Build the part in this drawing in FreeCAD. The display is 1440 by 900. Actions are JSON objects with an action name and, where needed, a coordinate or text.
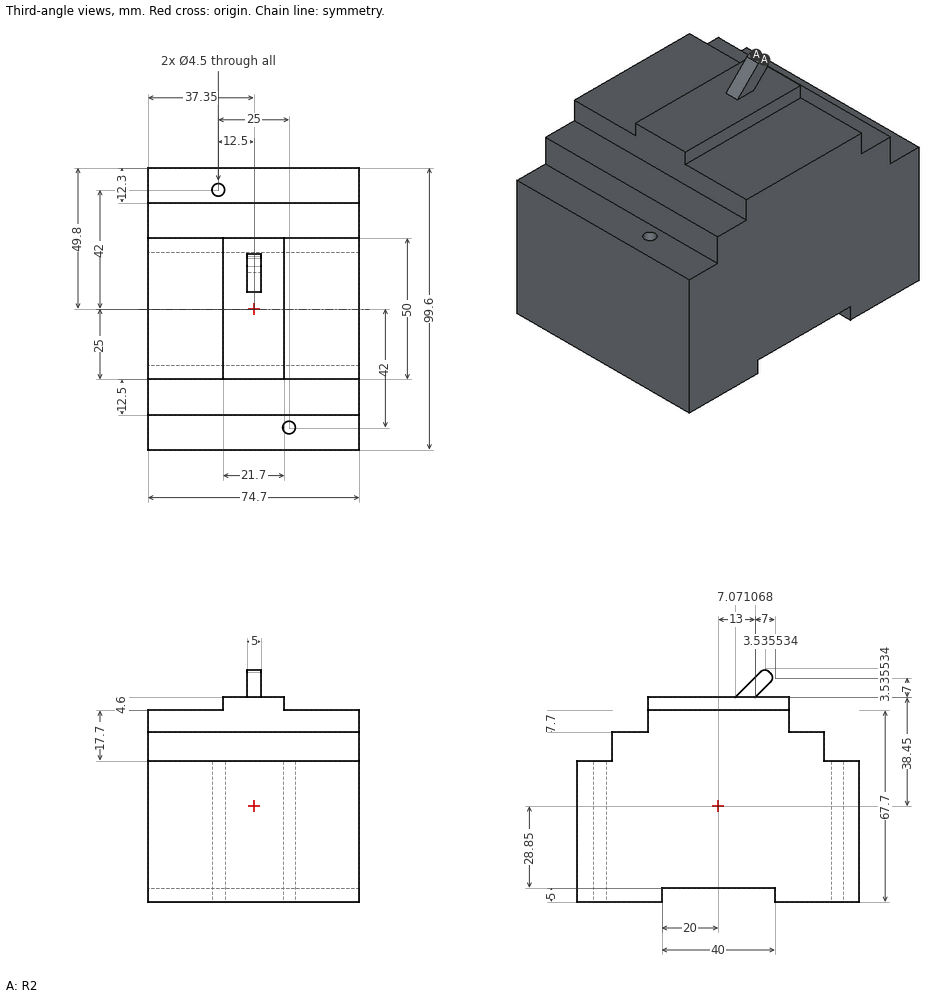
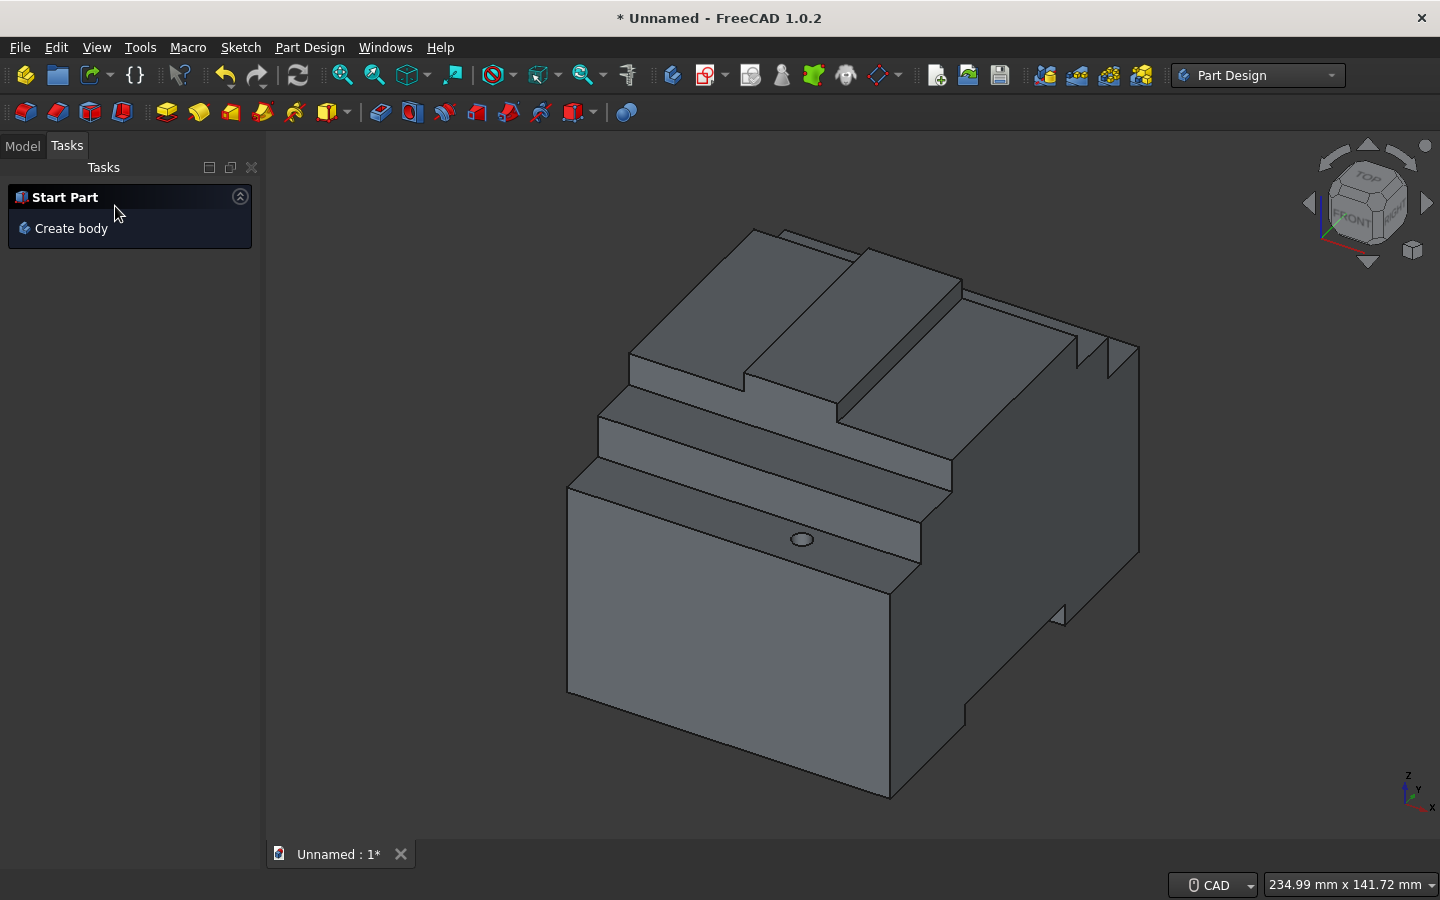
{"action": "left_click", "coordinate": [706, 76]}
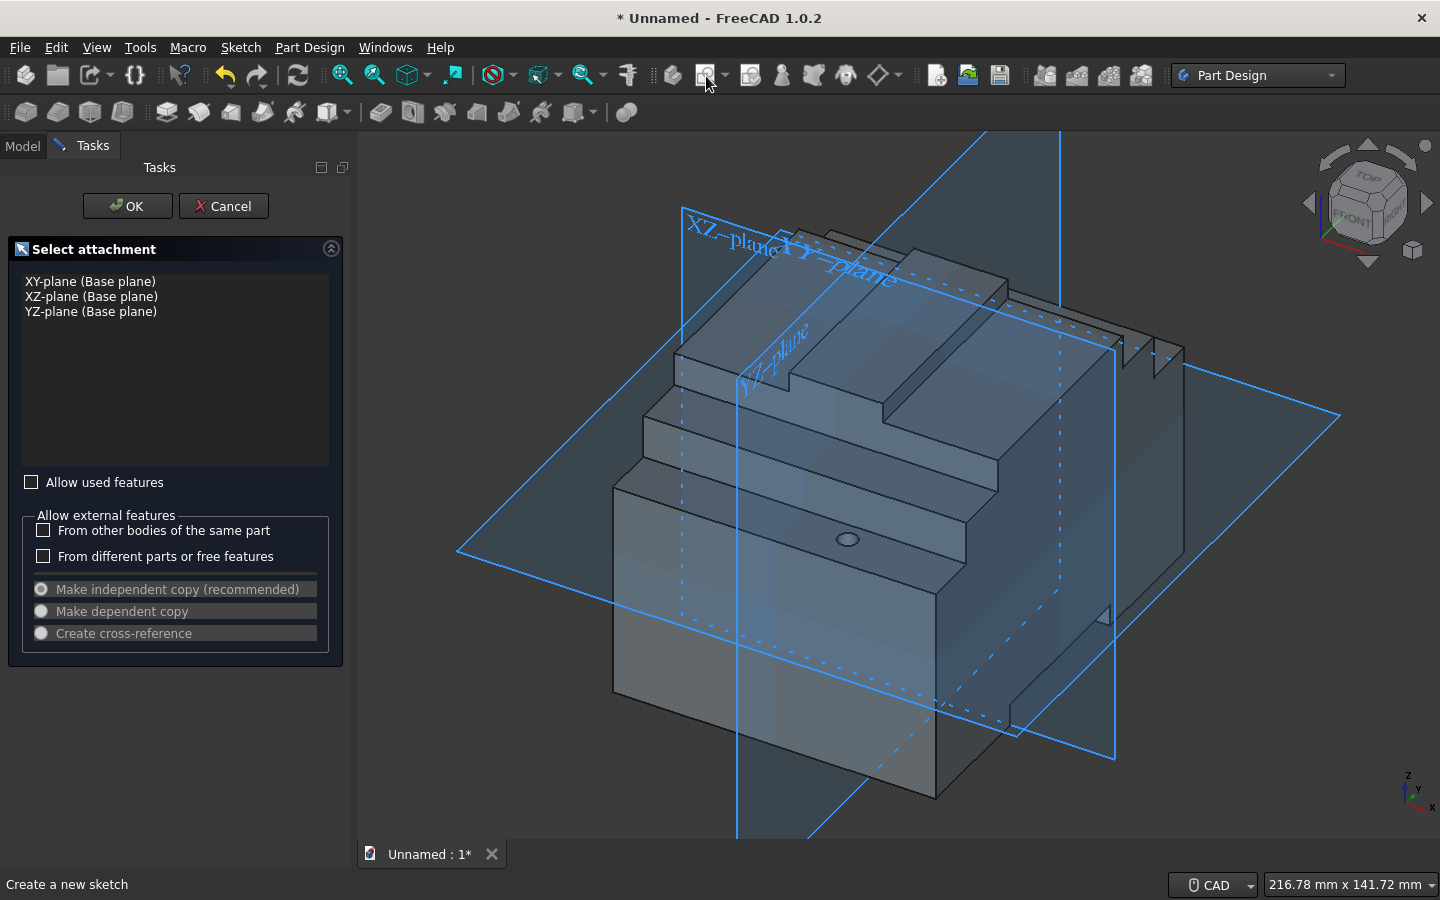
{"action": "left_click", "coordinate": [82, 312]}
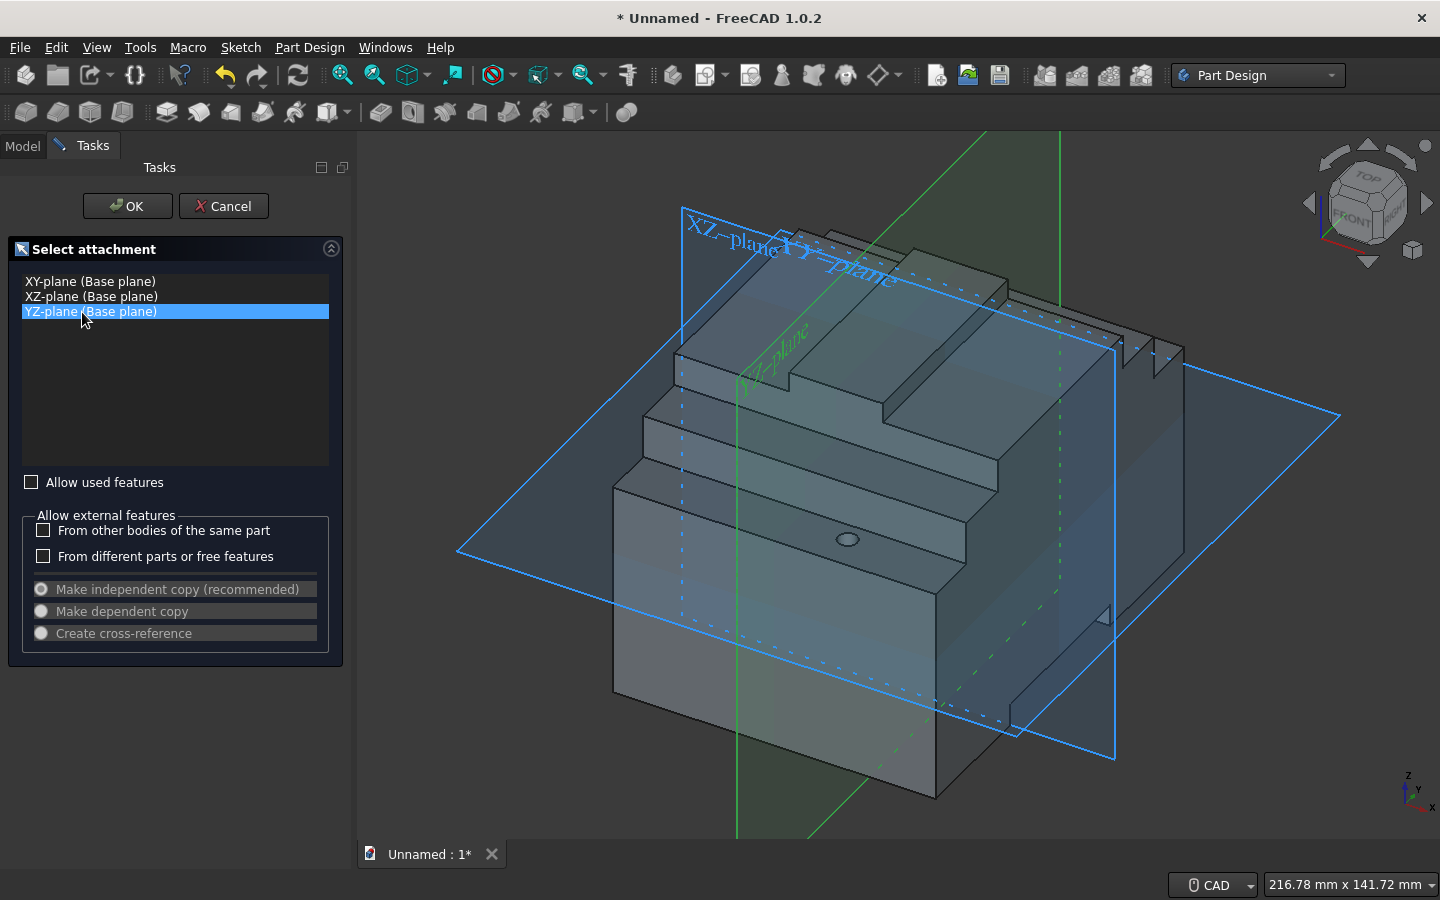
{"action": "left_click", "coordinate": [128, 206]}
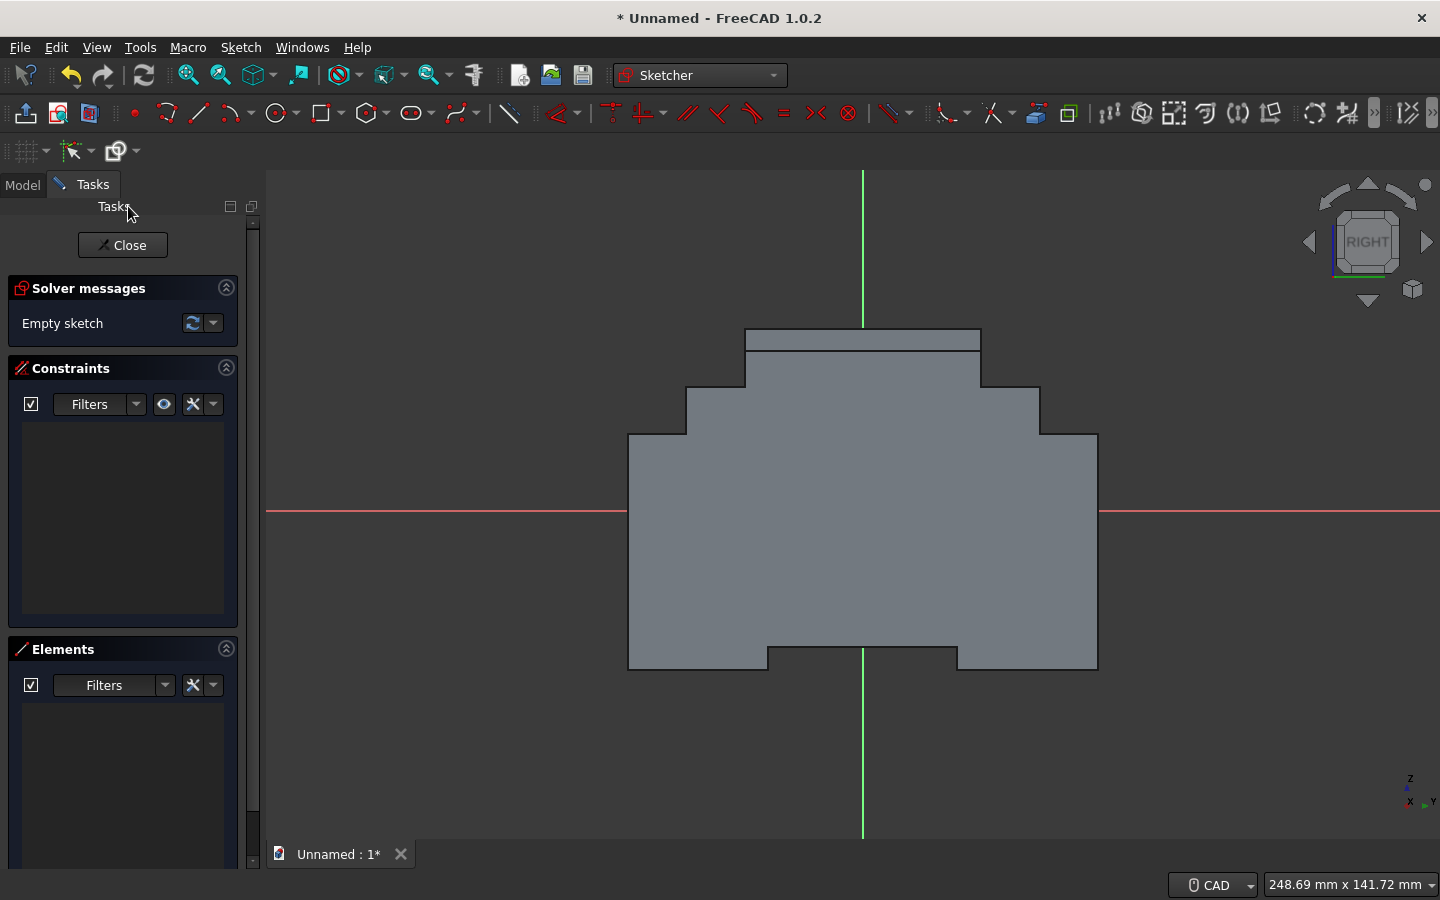
{"action": "left_click", "coordinate": [90, 114]}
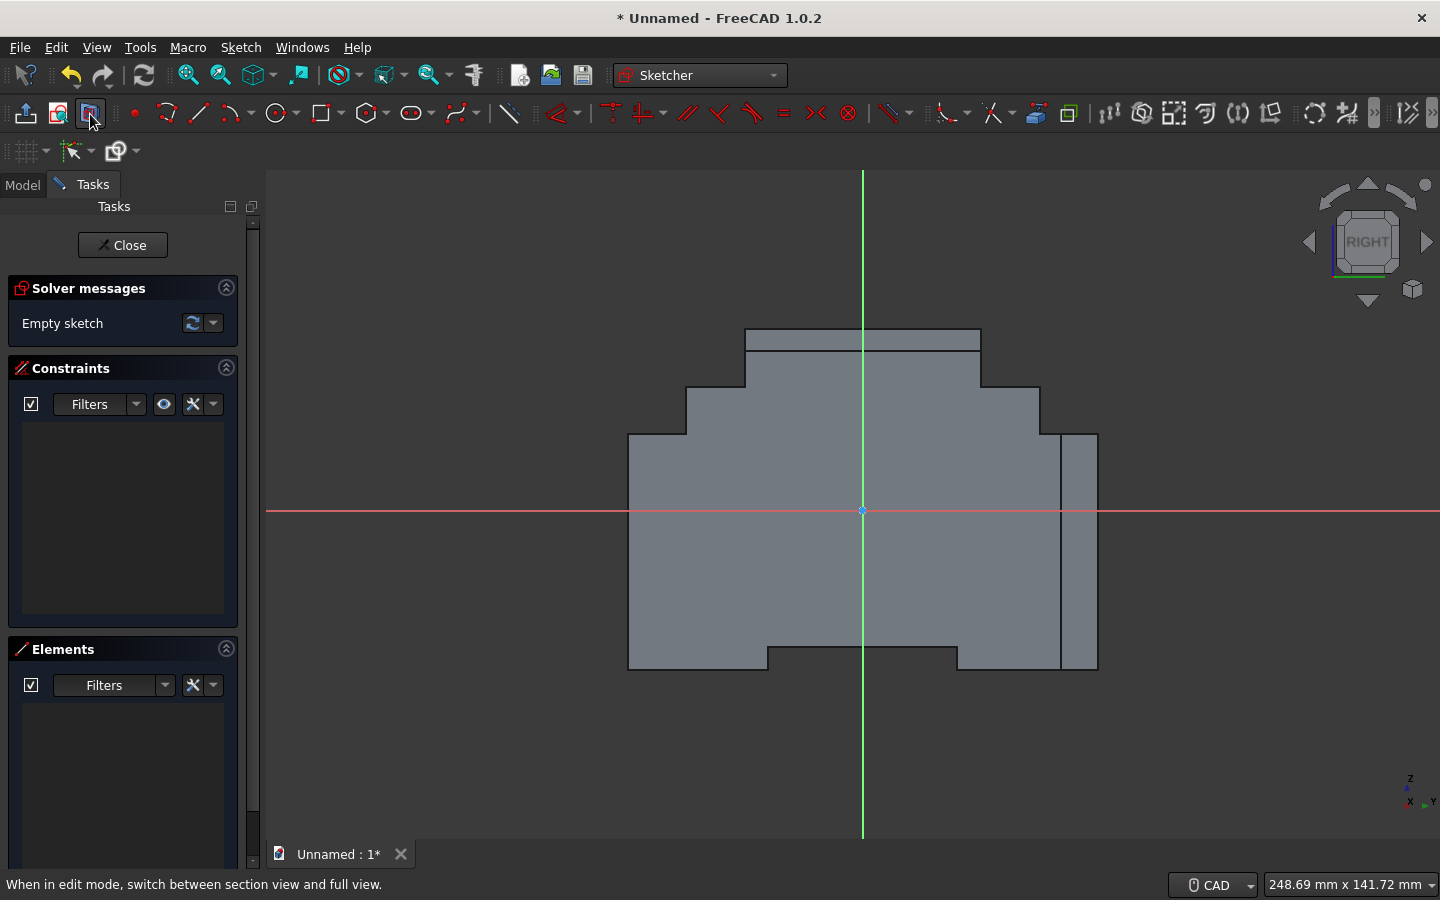
{"action": "scroll", "coordinate": [941, 279], "scroll_direction": "up", "scroll_amount": 11}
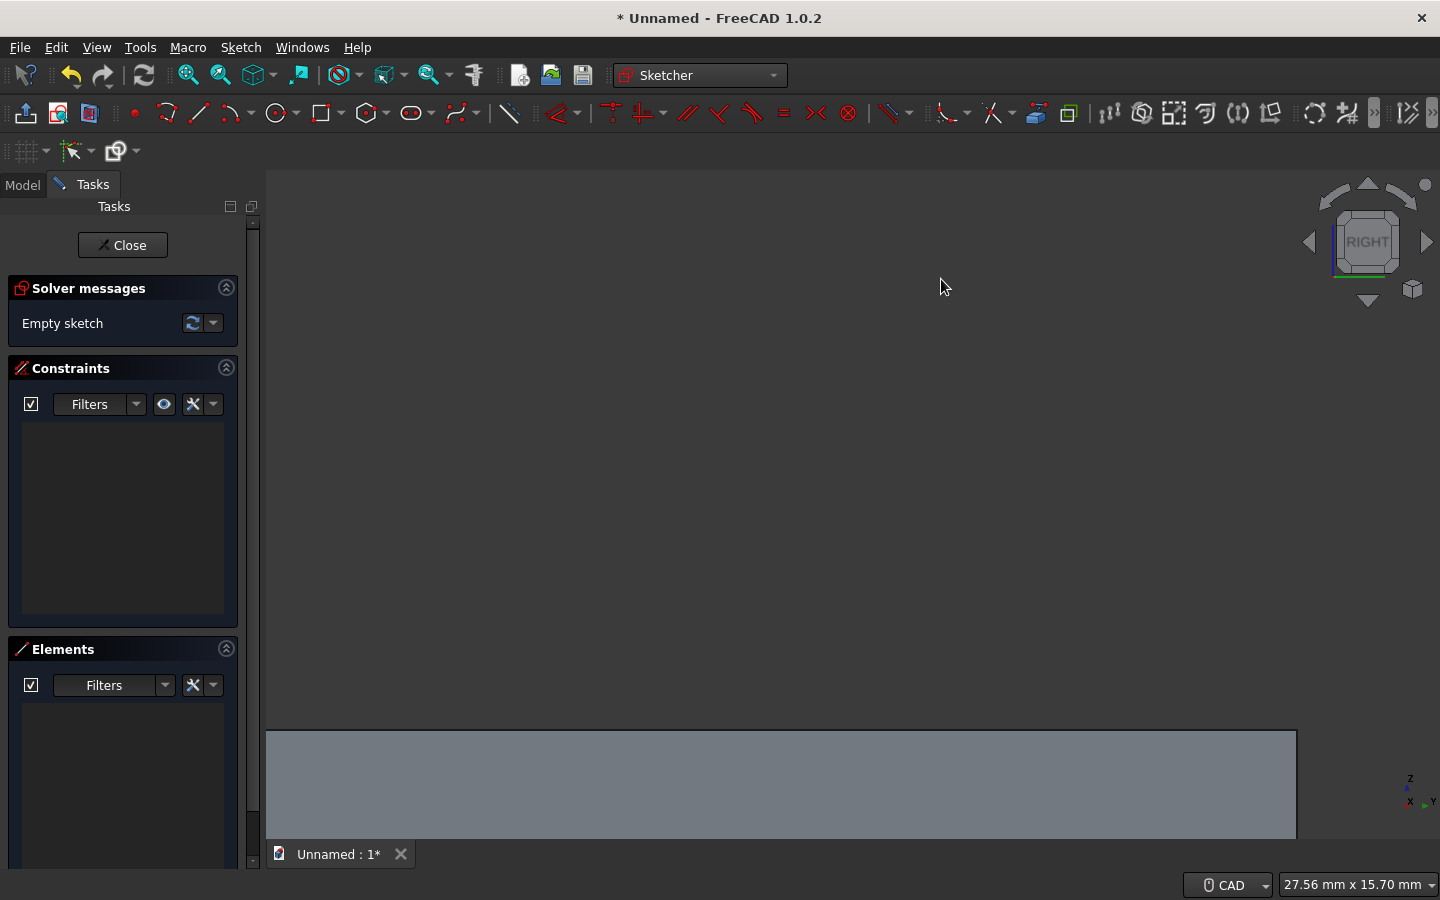
{"action": "left_click", "coordinate": [168, 114]}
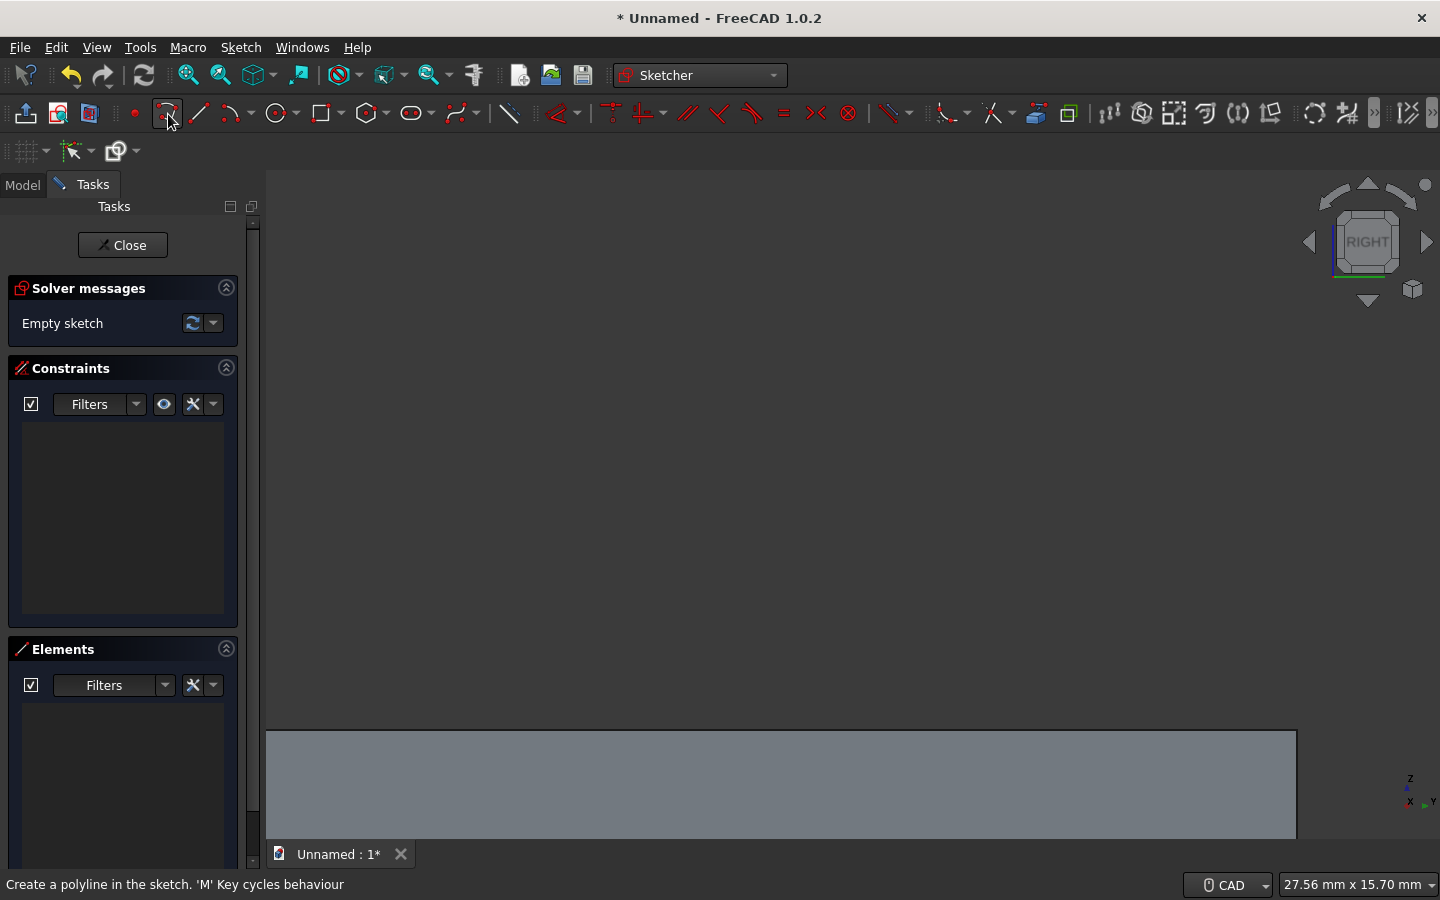
{"action": "left_click", "coordinate": [484, 730]}
{"action": "left_click", "coordinate": [785, 730]}
{"action": "left_click", "coordinate": [1084, 432]}
{"action": "left_click", "coordinate": [933, 282]}
{"action": "left_click", "coordinate": [484, 731]}
{"action": "key", "text": "Escape"}
{"action": "key", "text": "Escape"}